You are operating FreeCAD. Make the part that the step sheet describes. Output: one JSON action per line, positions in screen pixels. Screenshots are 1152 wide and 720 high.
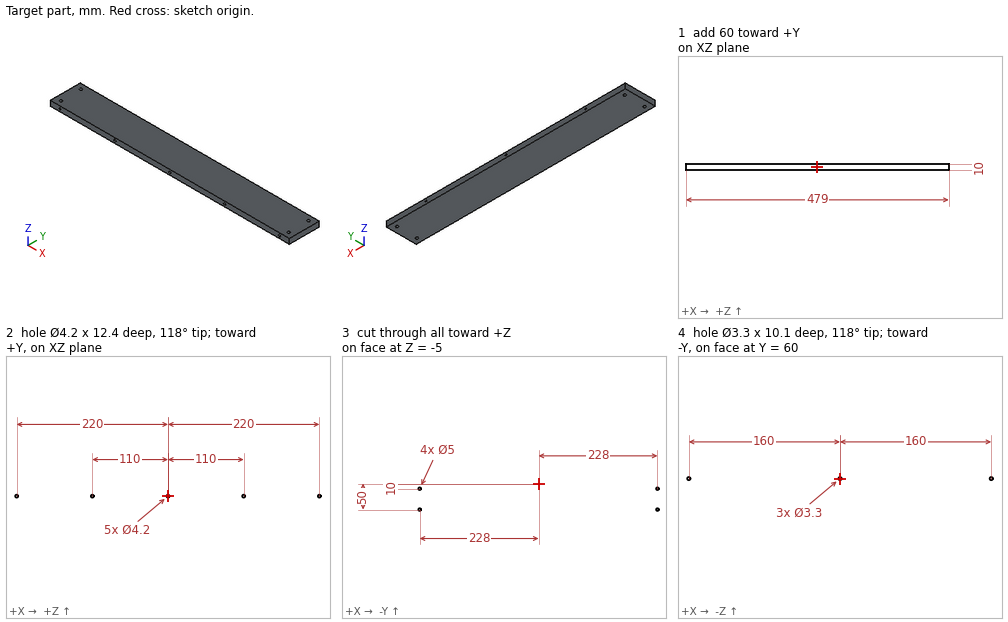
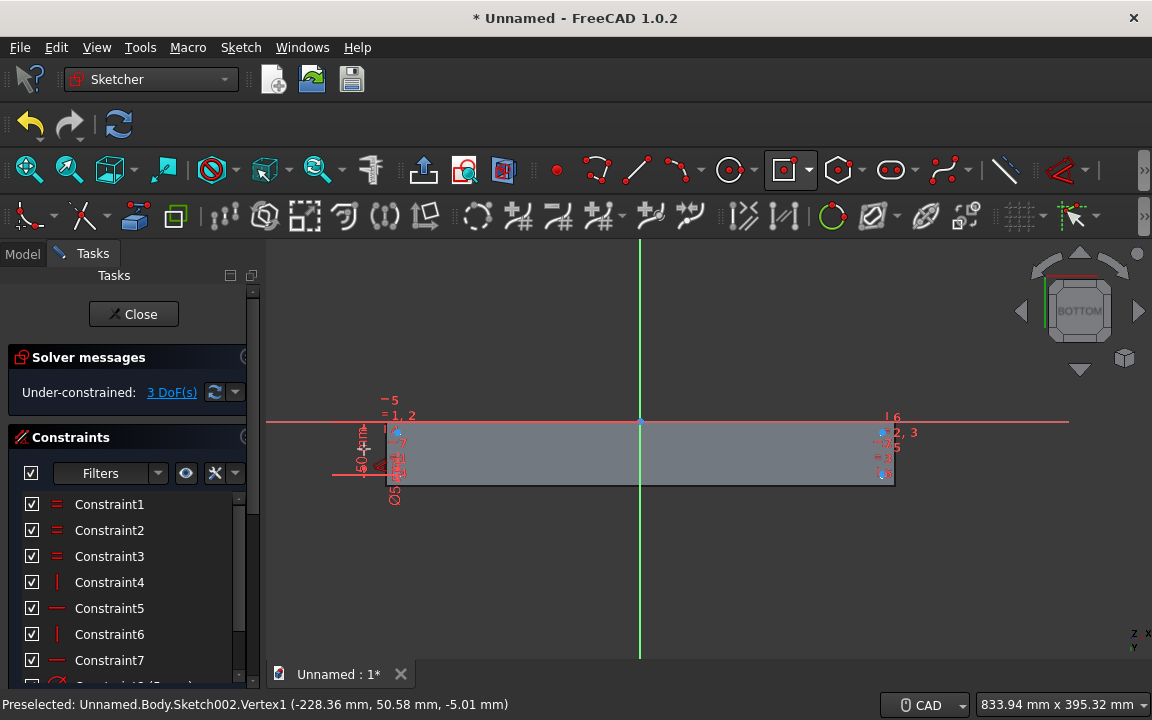
{"action": "scroll", "coordinate": [398, 433], "scroll_direction": "up", "scroll_amount": 7}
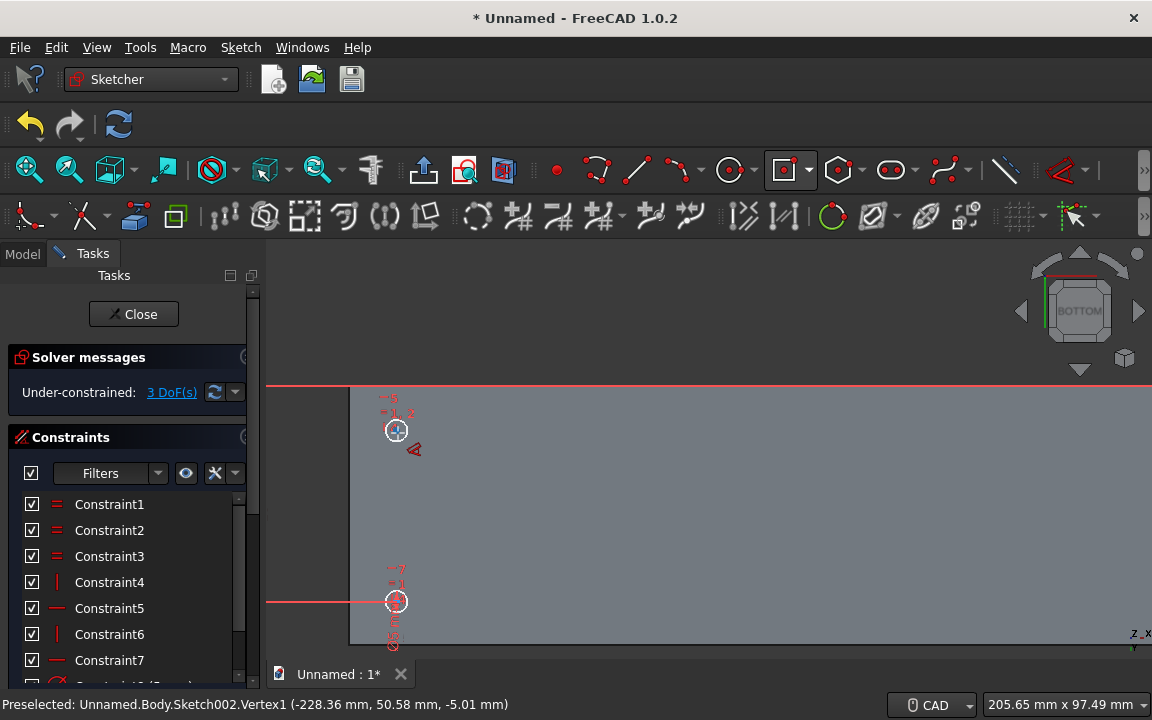
{"action": "left_click", "coordinate": [397, 431]}
{"action": "left_click", "coordinate": [363, 408]}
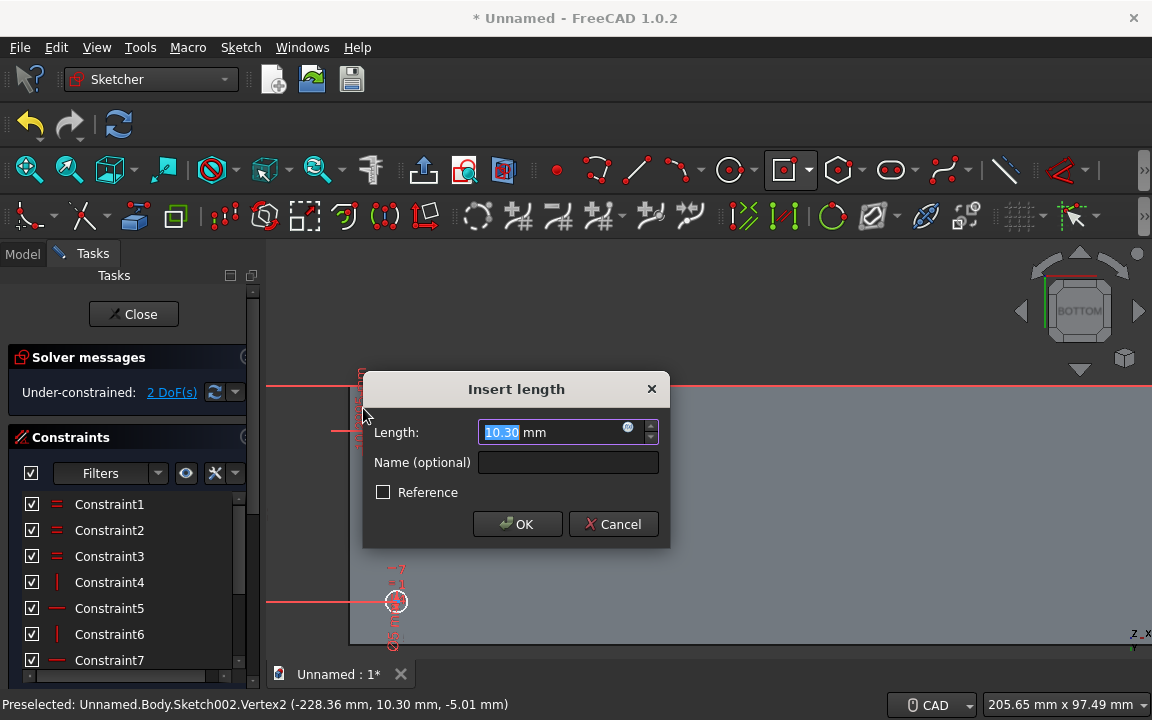
{"action": "type", "text": "10"}
{"action": "key", "text": "Return"}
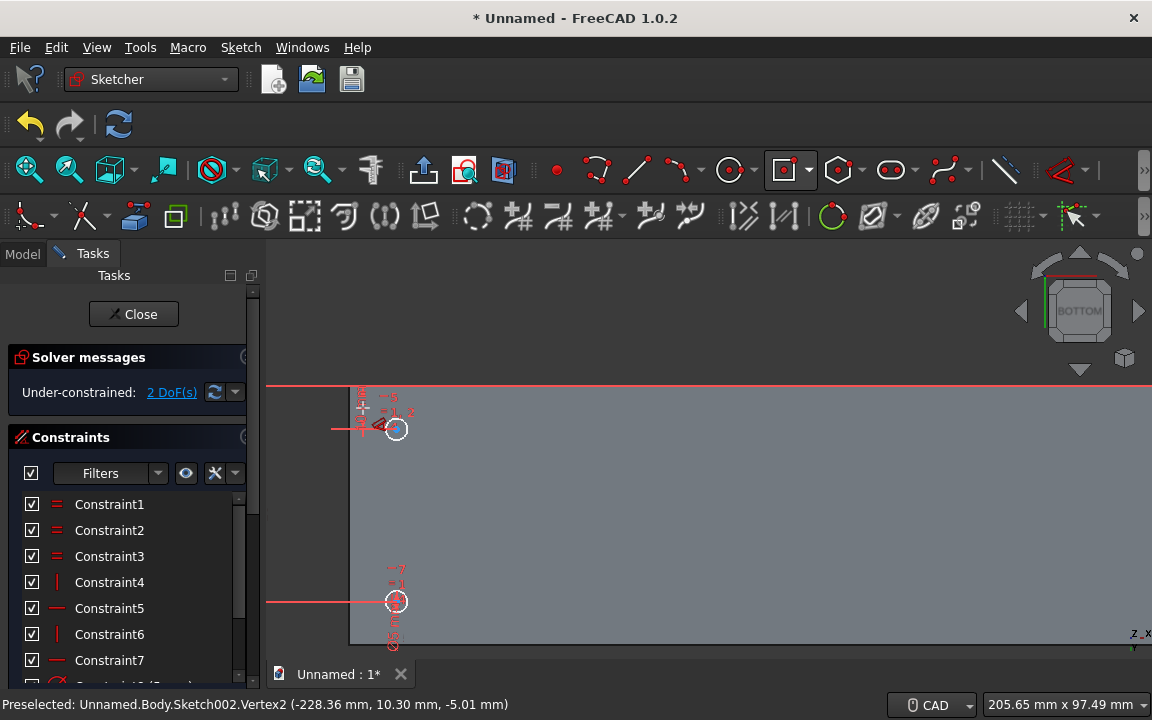
{"action": "scroll", "coordinate": [398, 433], "scroll_direction": "down", "scroll_amount": 7}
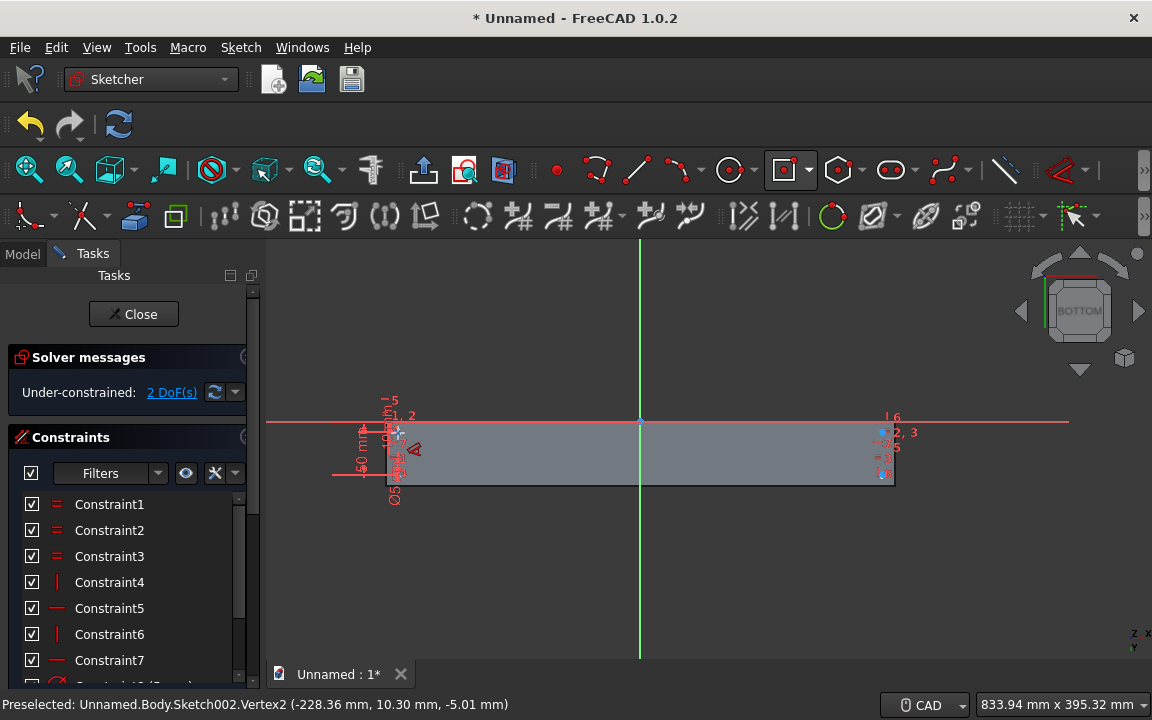
{"action": "left_click", "coordinate": [398, 475]}
{"action": "left_click", "coordinate": [519, 388]}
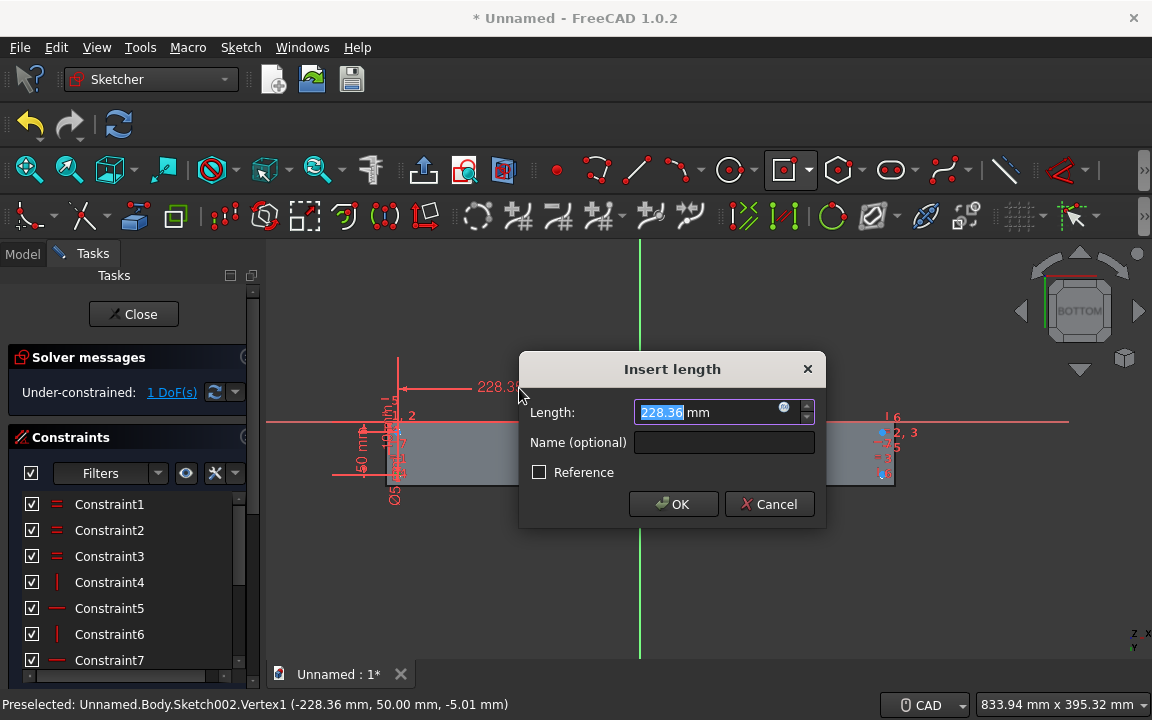
{"action": "type", "text": "228"}
{"action": "key", "text": "Return"}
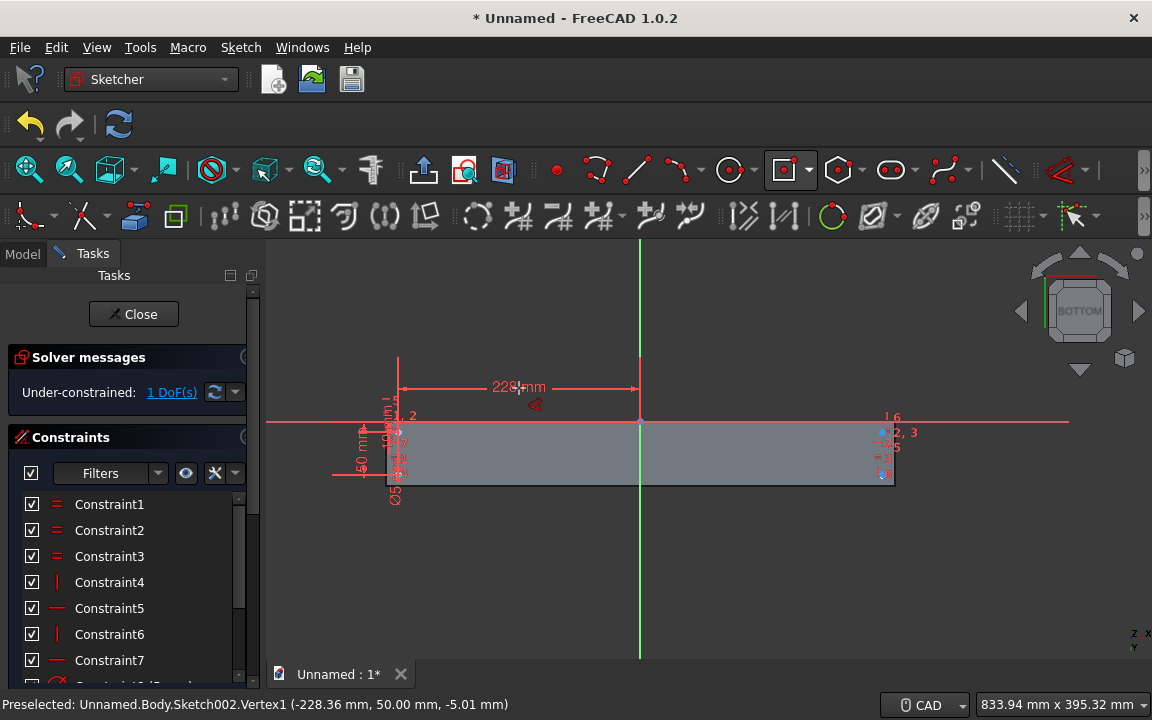
{"action": "left_click", "coordinate": [882, 432]}
{"action": "left_click", "coordinate": [761, 388]}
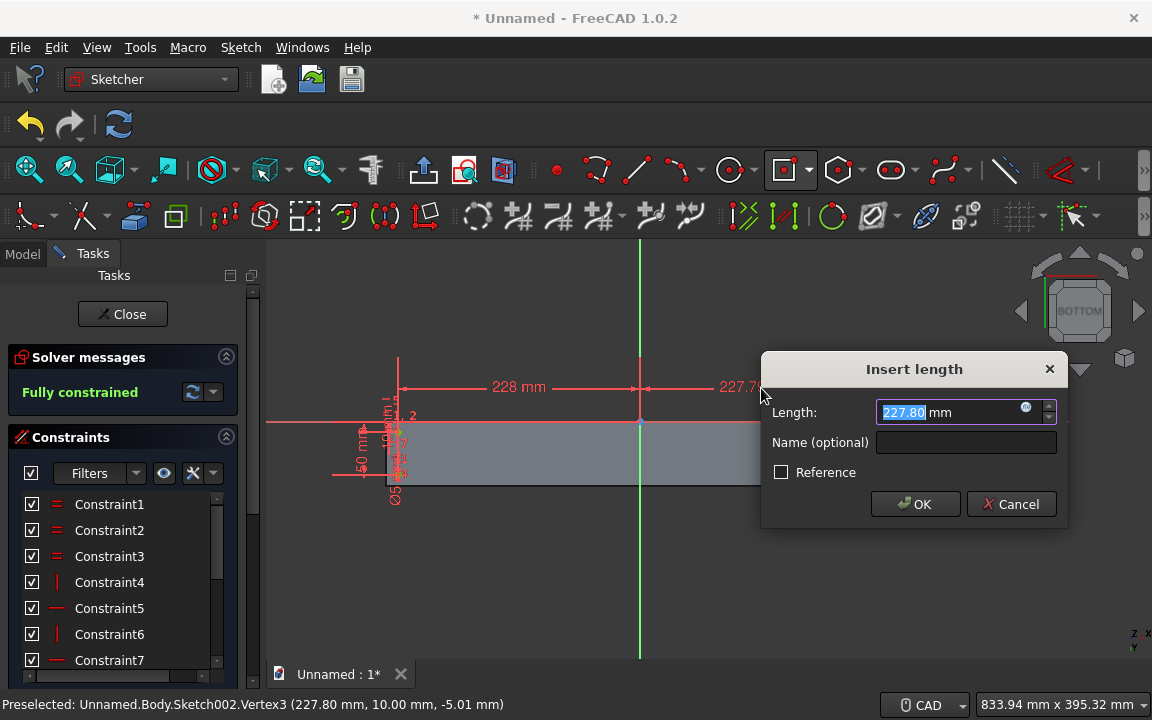
{"action": "type", "text": "228"}
{"action": "key", "text": "Return"}
{"action": "key", "text": "Escape"}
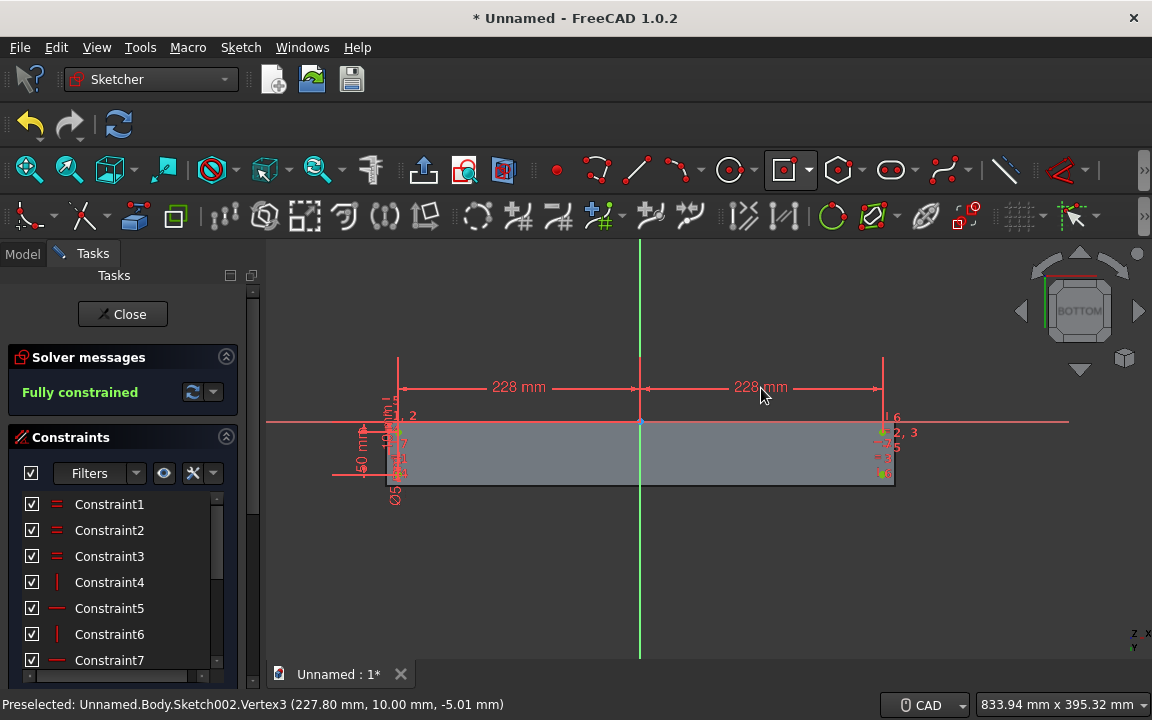
{"action": "left_click", "coordinate": [123, 314]}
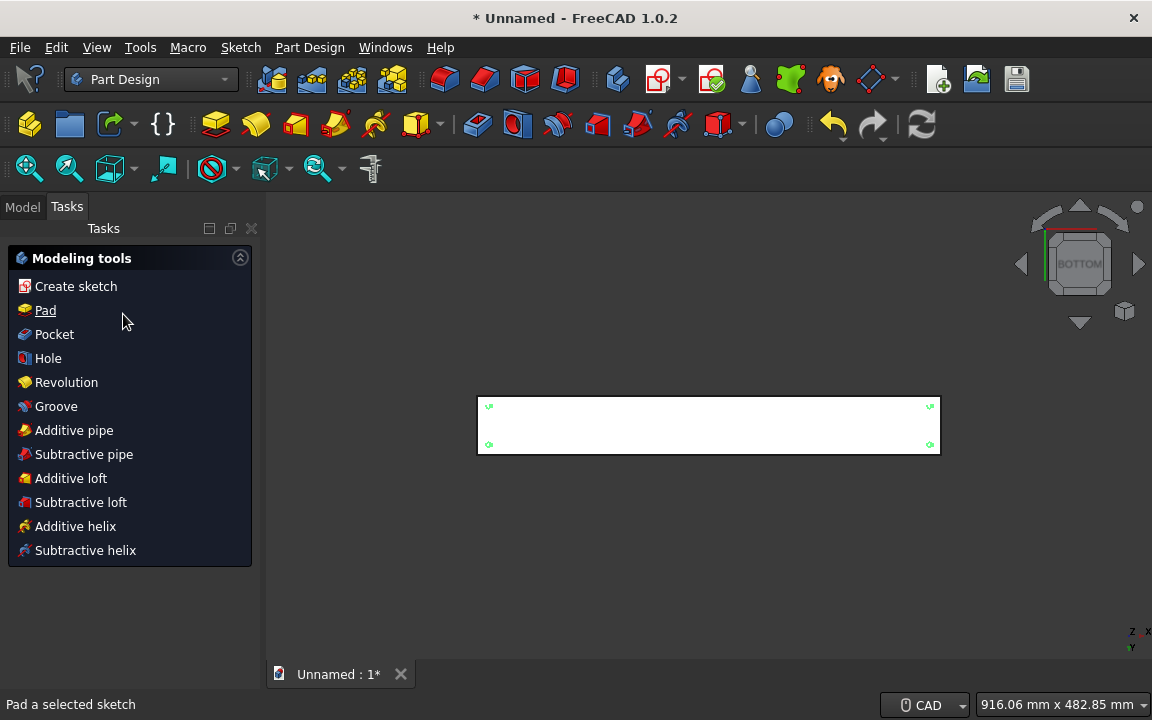
{"action": "left_click", "coordinate": [478, 124]}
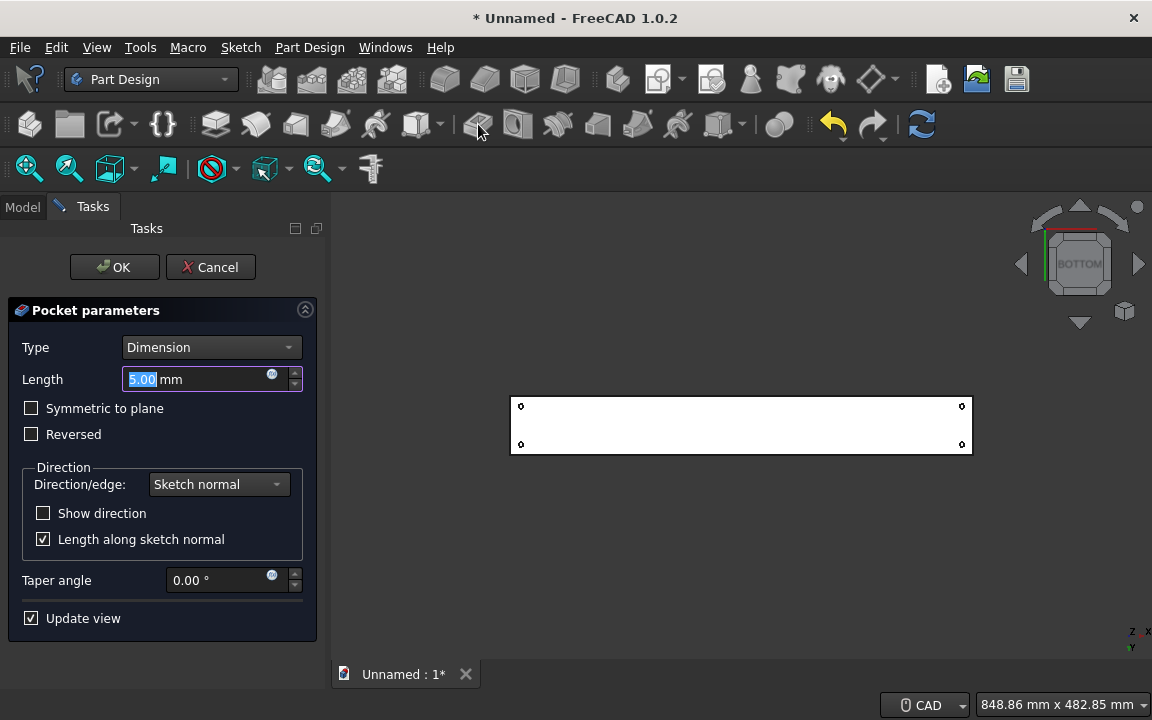
{"action": "left_click", "coordinate": [212, 348]}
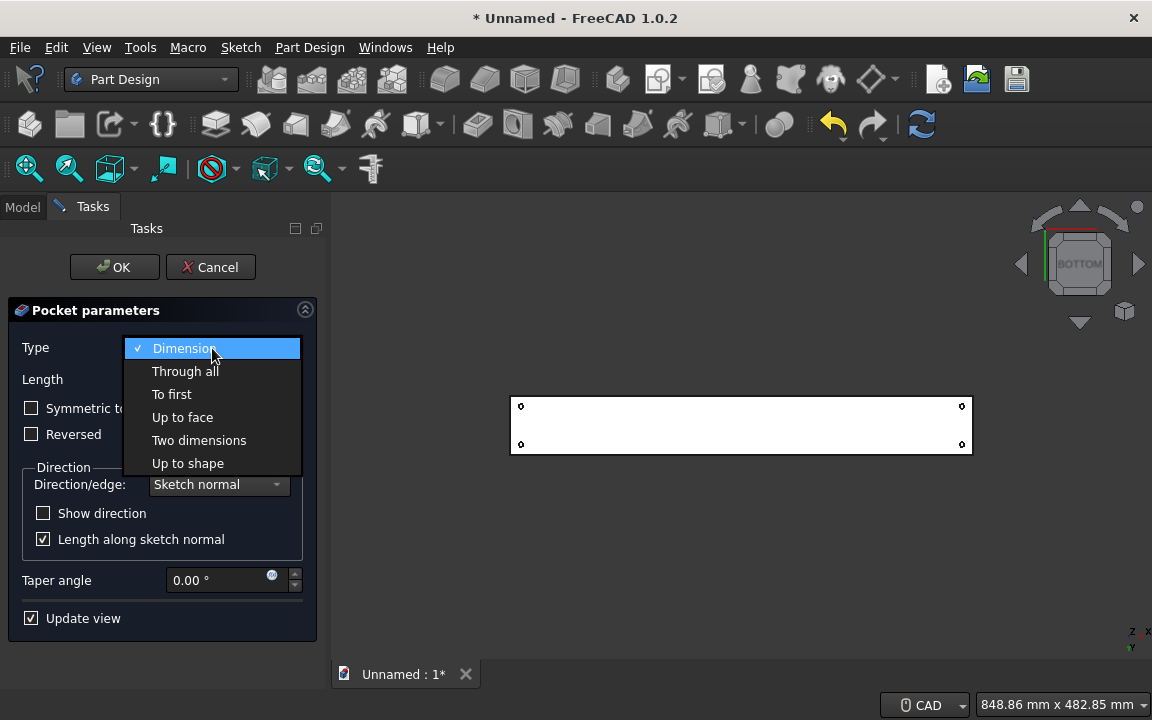
{"action": "left_click", "coordinate": [212, 372]}